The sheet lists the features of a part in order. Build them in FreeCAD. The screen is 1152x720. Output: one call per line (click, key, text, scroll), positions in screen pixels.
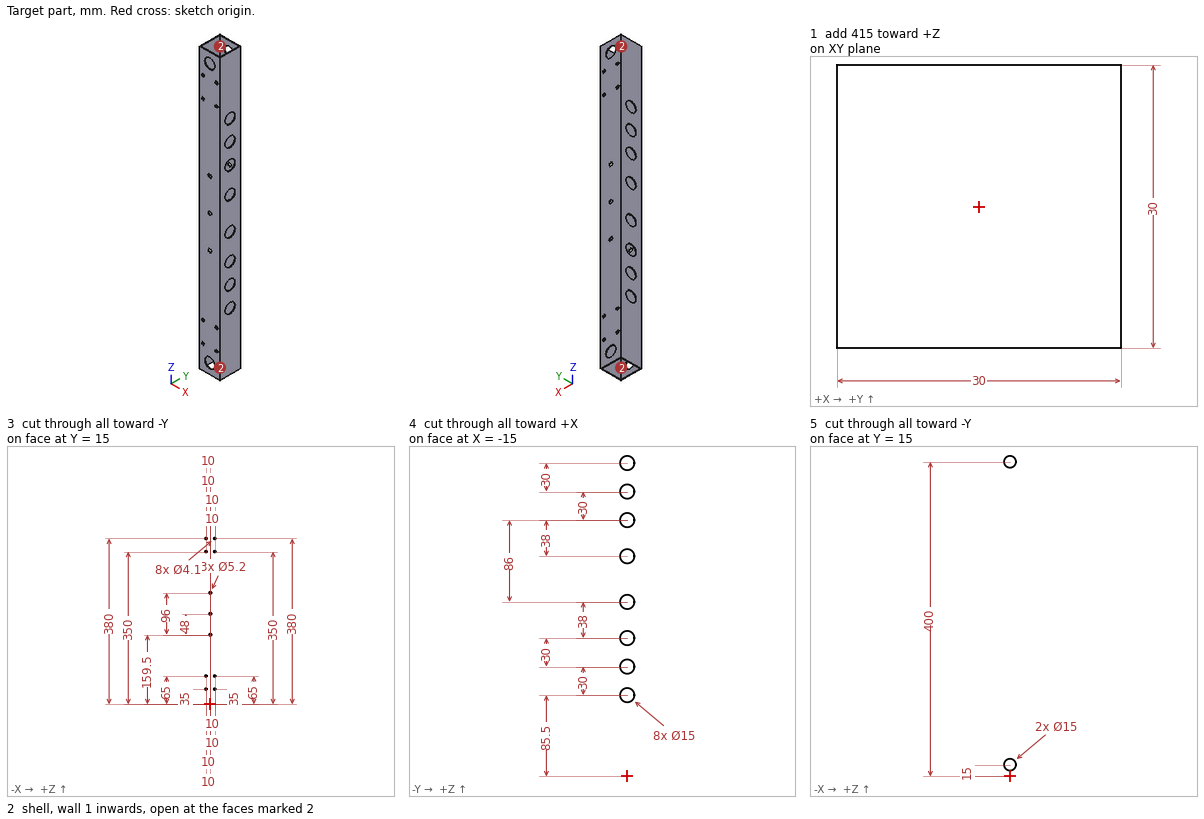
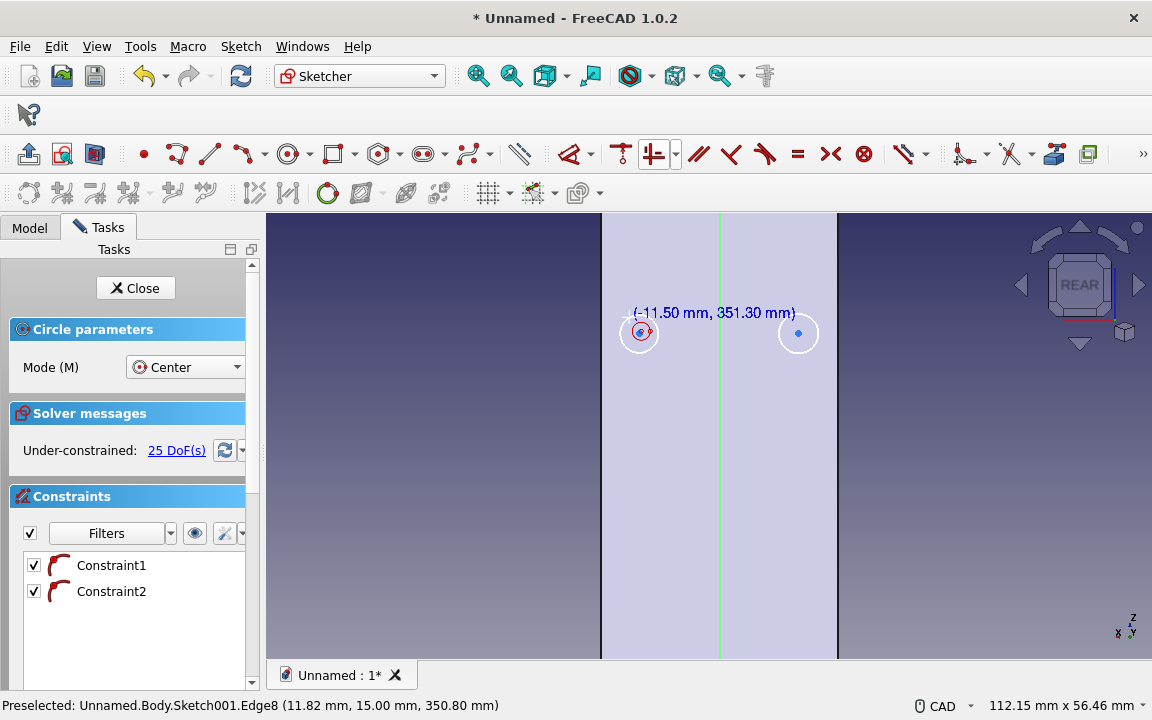
scroll(633, 321, down, 12)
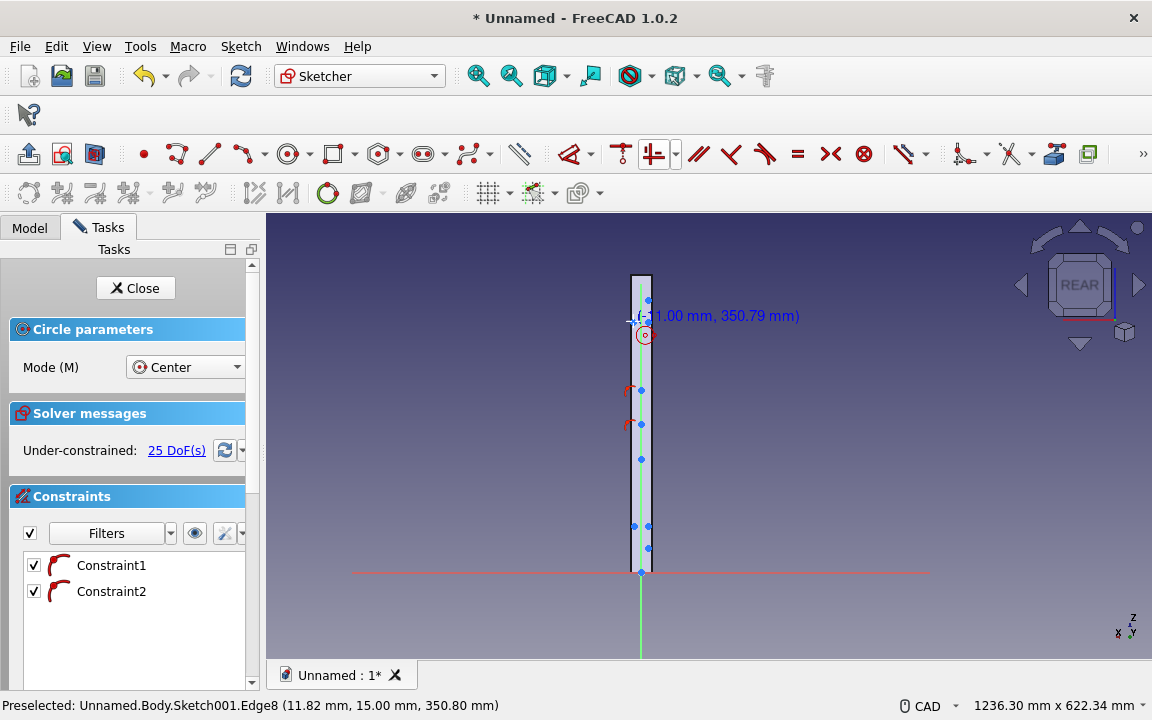
scroll(634, 548, up, 14)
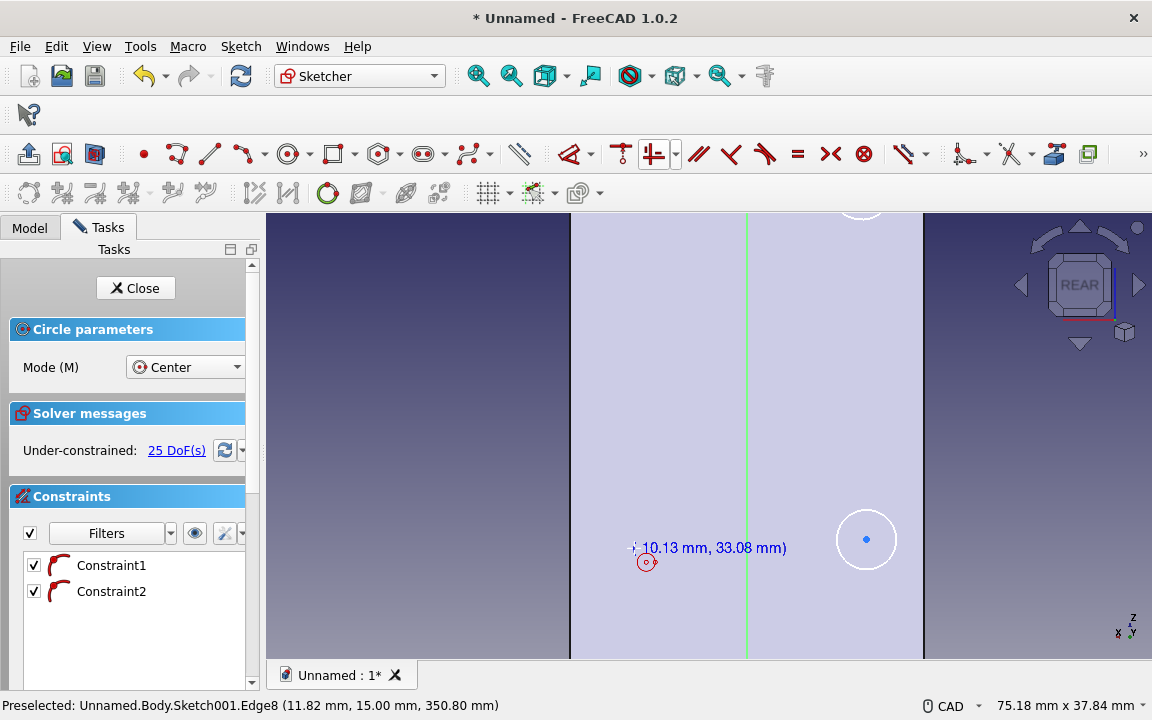
scroll(634, 549, down, 14)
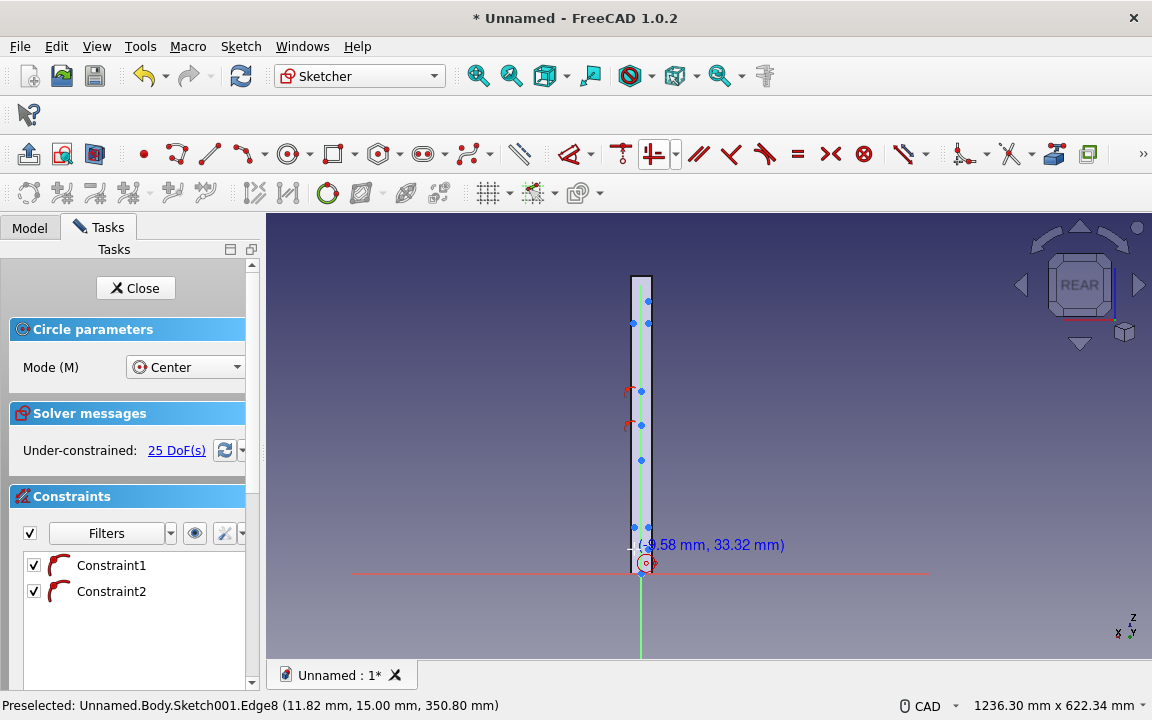
scroll(634, 549, up, 4)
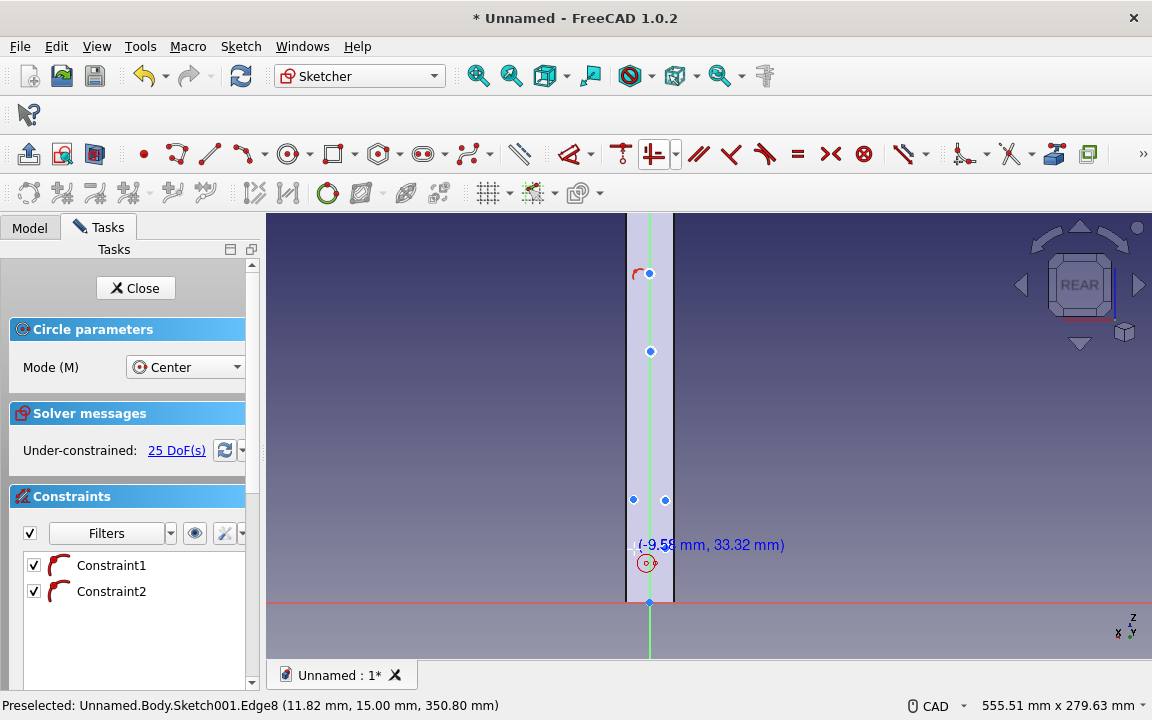
click(634, 547)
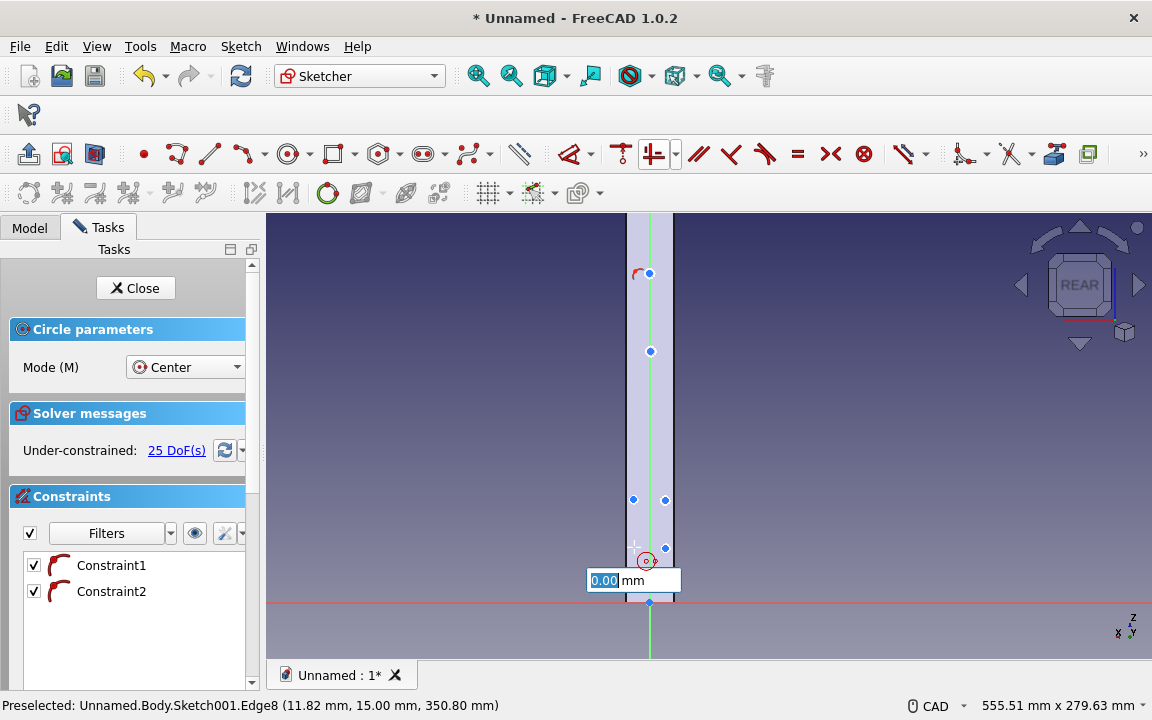
scroll(631, 545, up, 8)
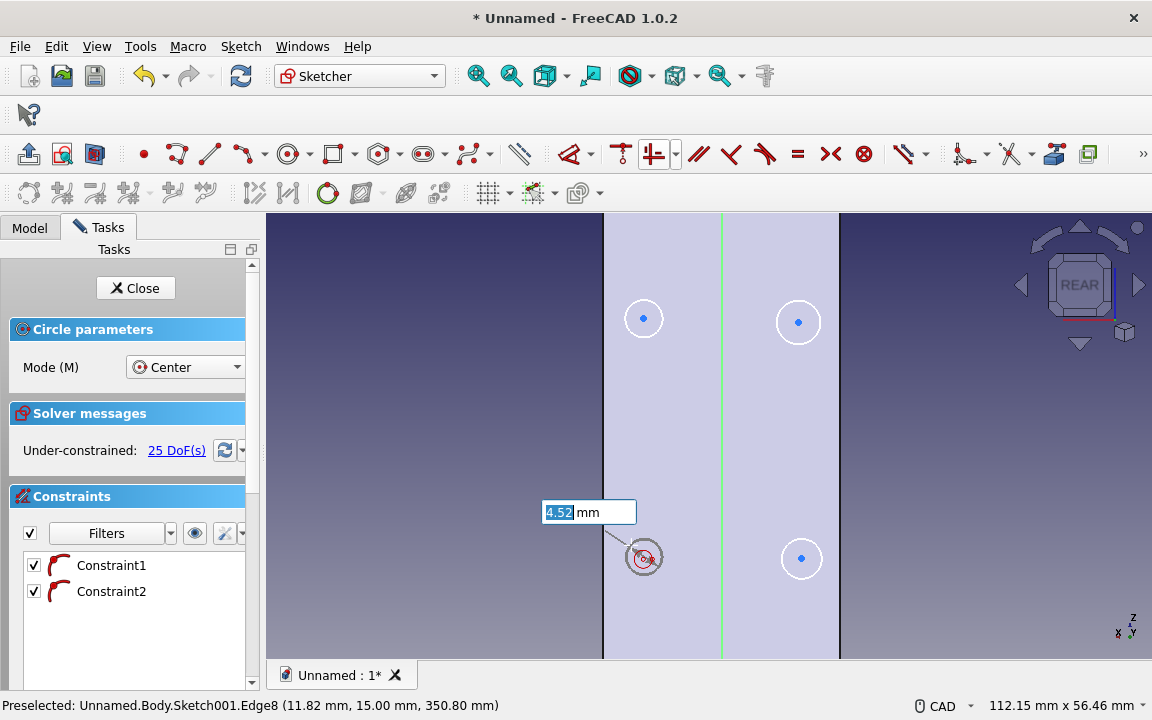
click(631, 541)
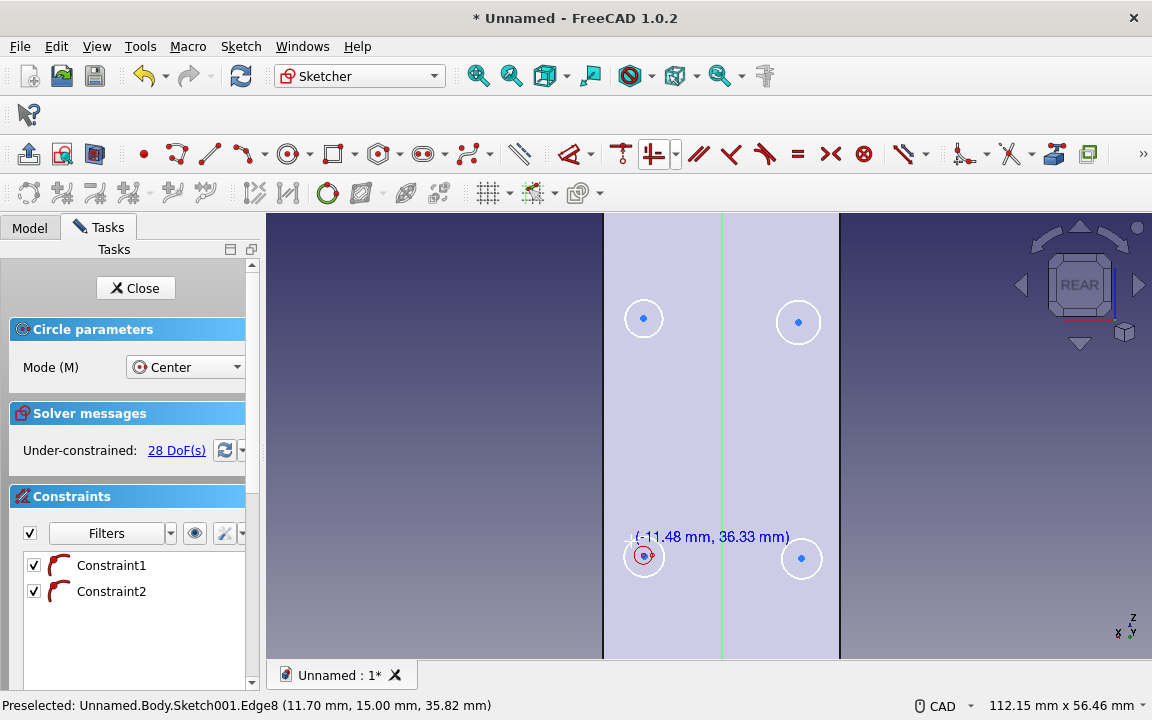
scroll(632, 547, down, 12)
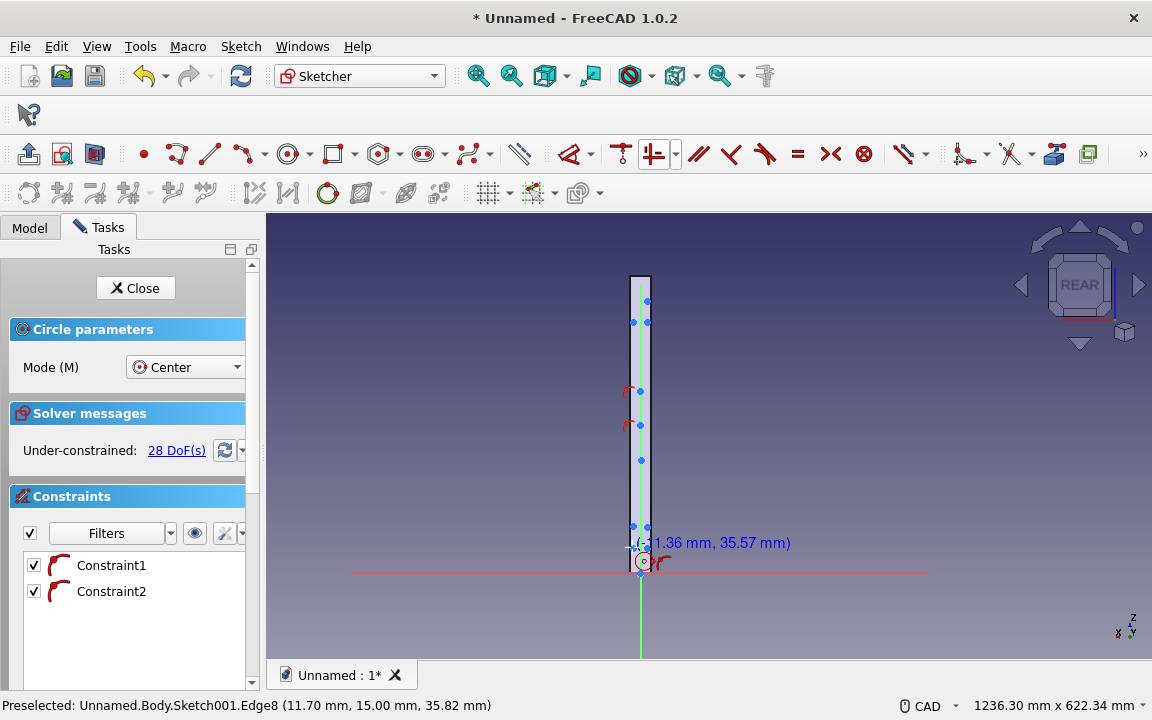
scroll(633, 301, up, 14)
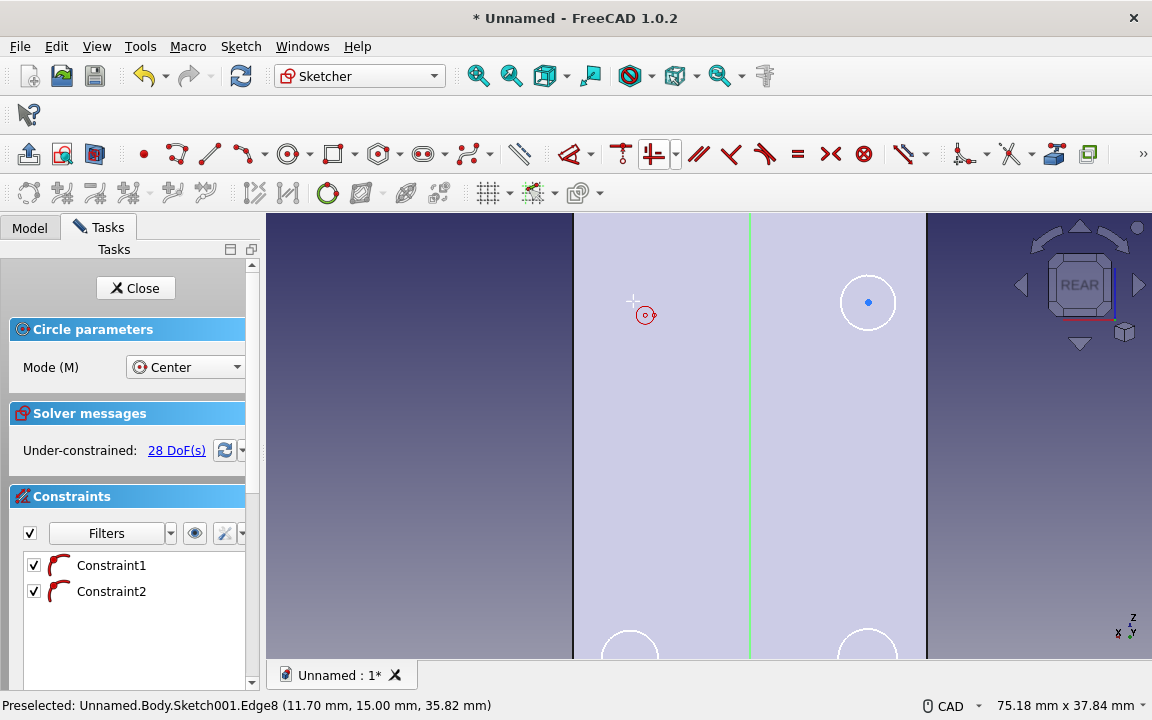
scroll(633, 301, down, 14)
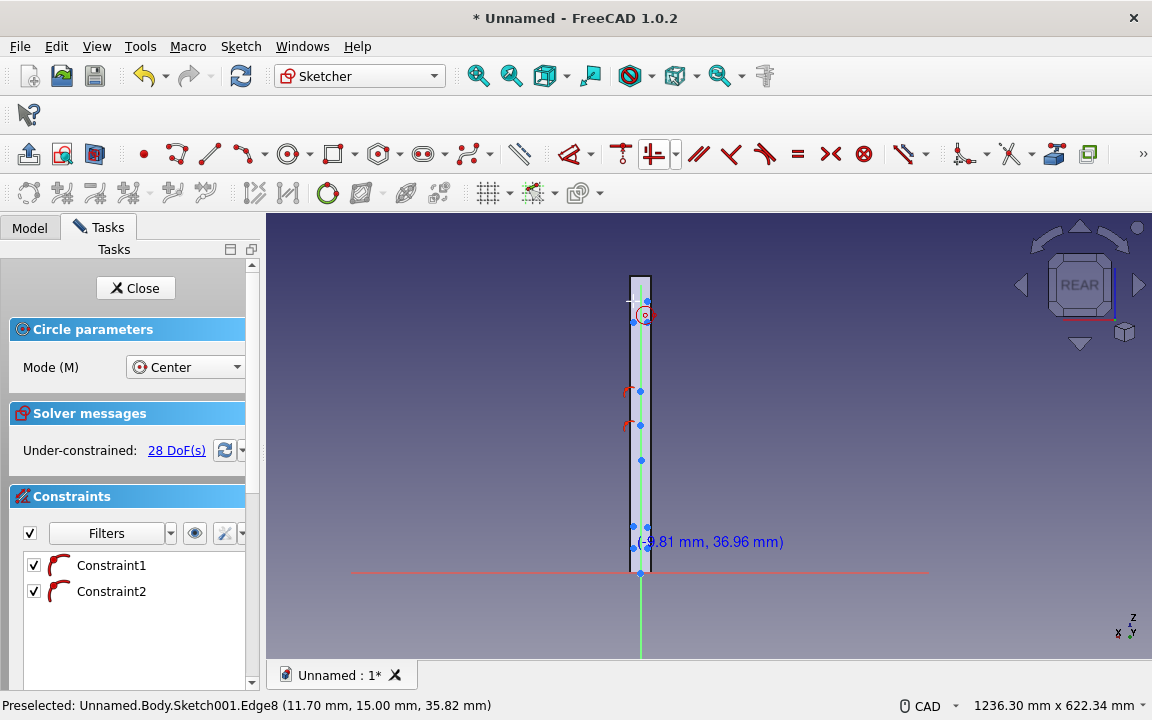
scroll(633, 301, up, 4)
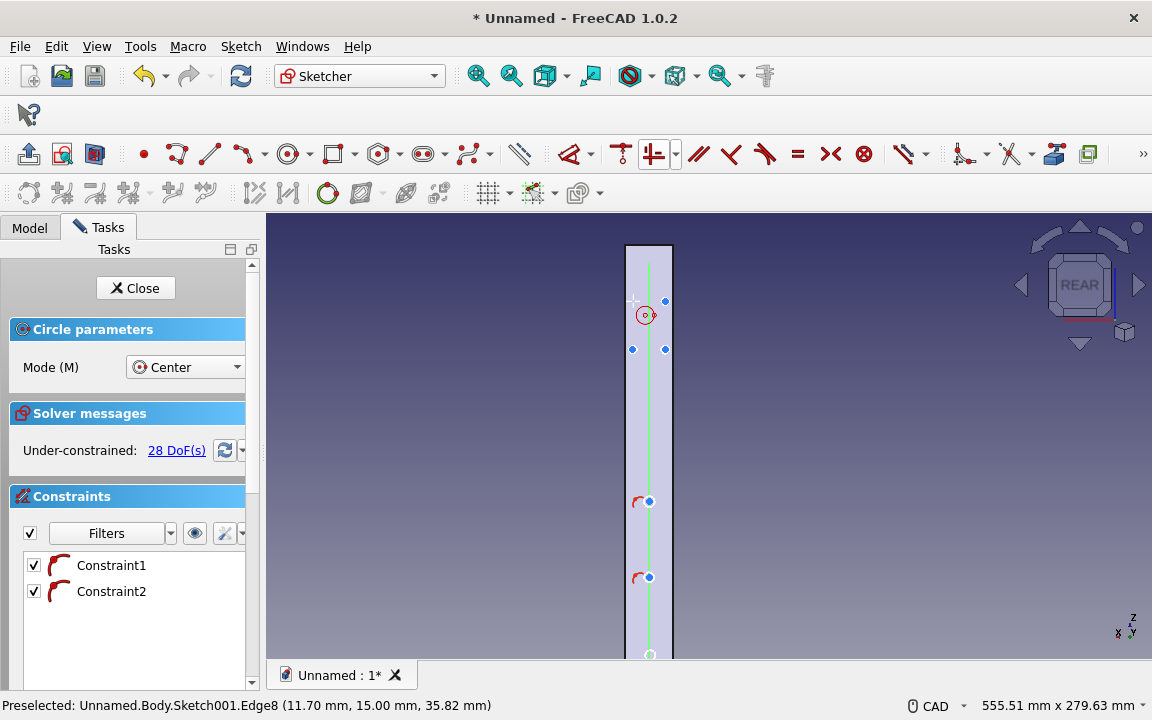
click(633, 301)